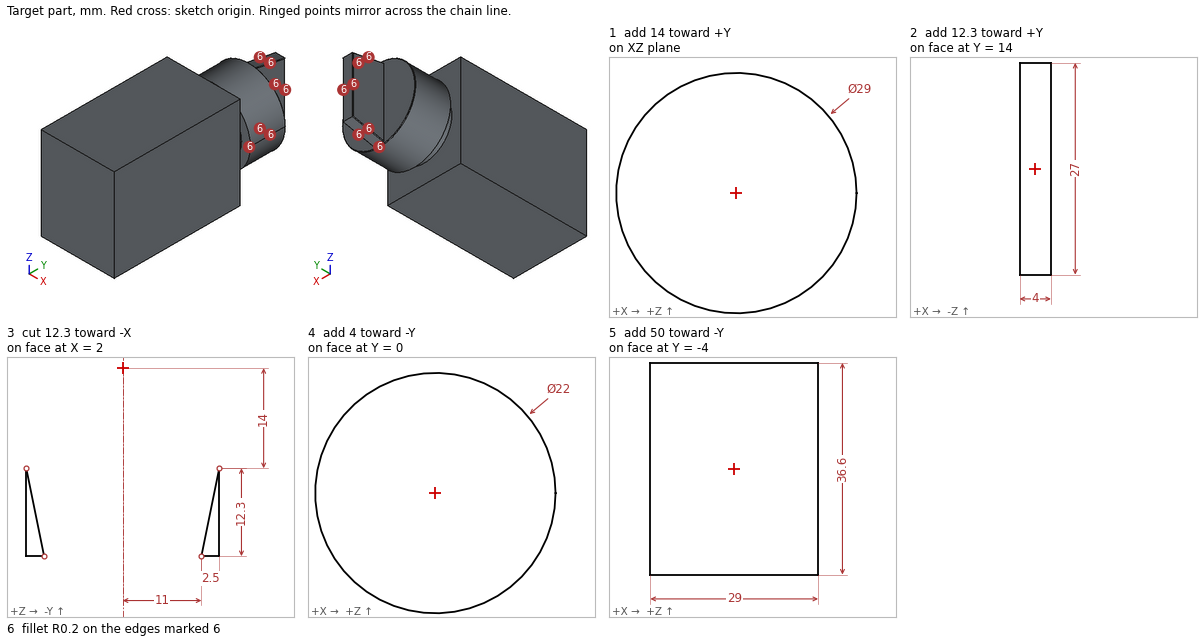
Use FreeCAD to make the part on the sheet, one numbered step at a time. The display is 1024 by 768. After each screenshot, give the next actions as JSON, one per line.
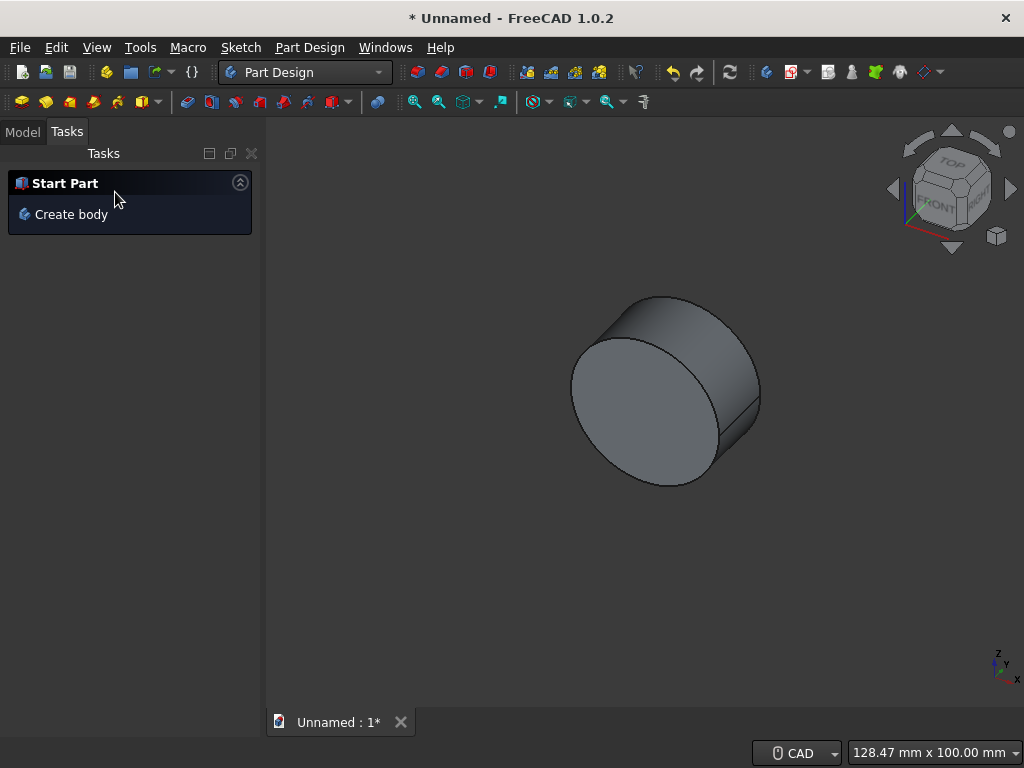
{"action": "left_click", "coordinate": [416, 102]}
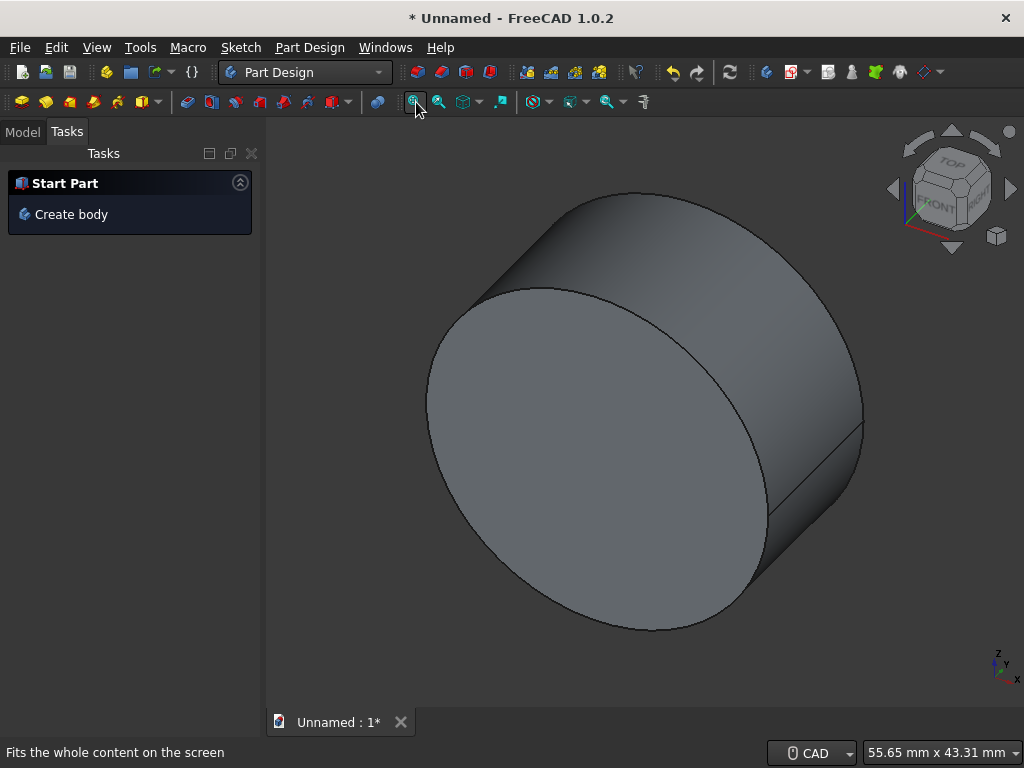
{"action": "key", "text": "4"}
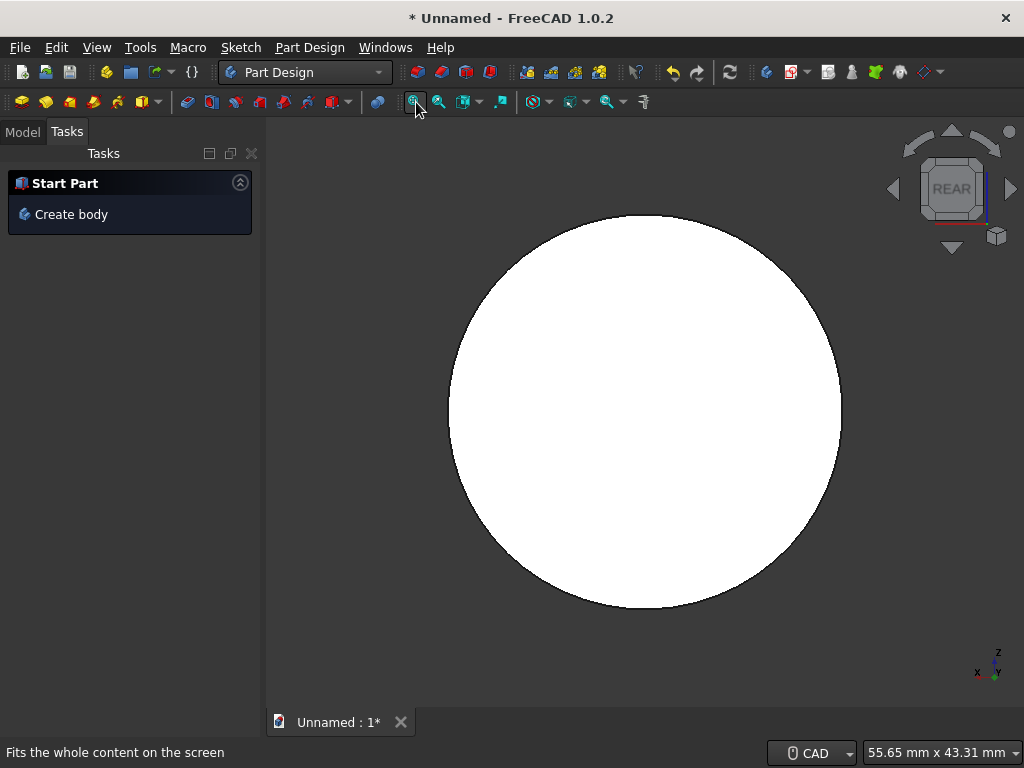
{"action": "left_click", "coordinate": [645, 411]}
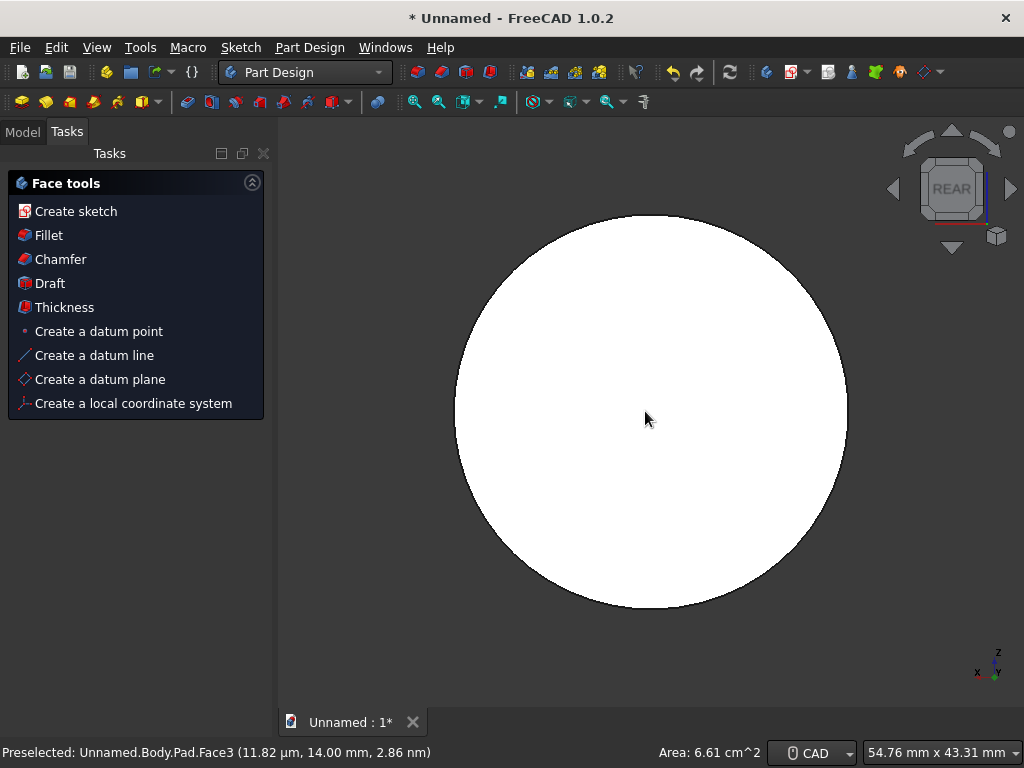
{"action": "left_click", "coordinate": [792, 72]}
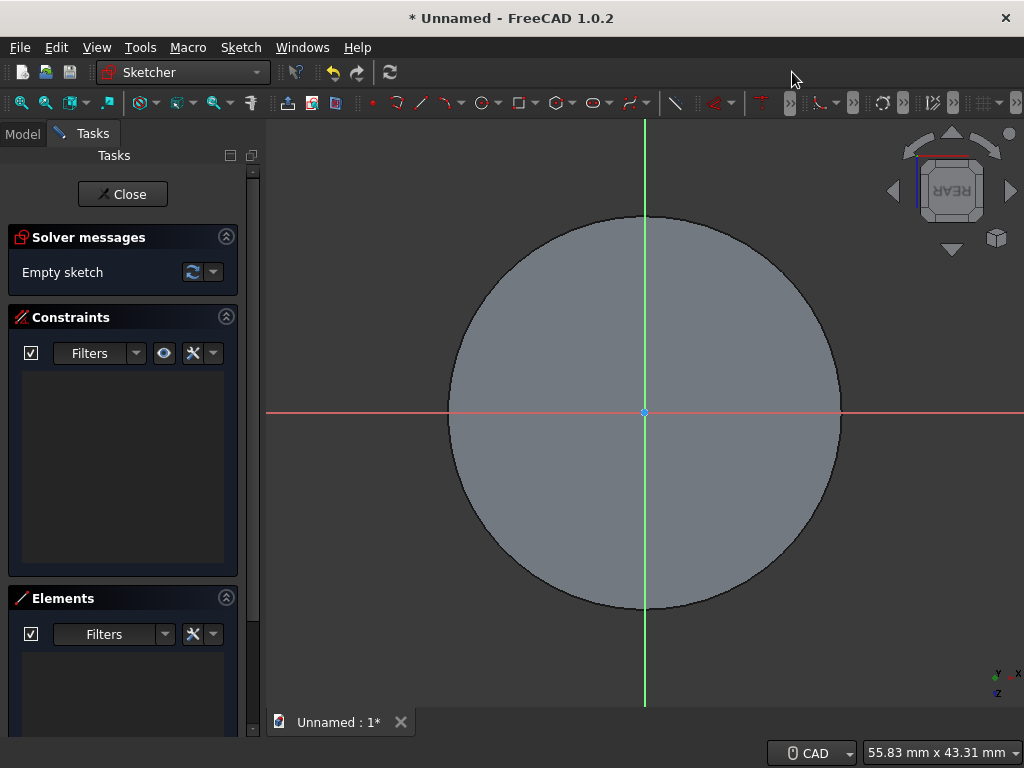
{"action": "left_click", "coordinate": [538, 104]}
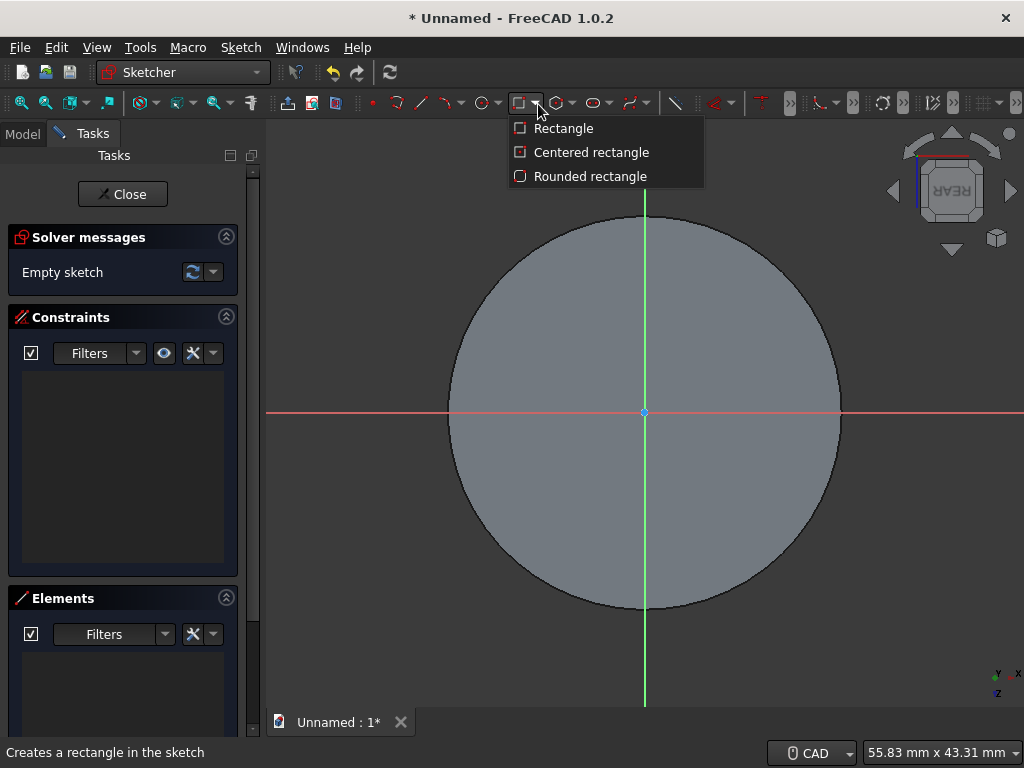
{"action": "left_click", "coordinate": [606, 152]}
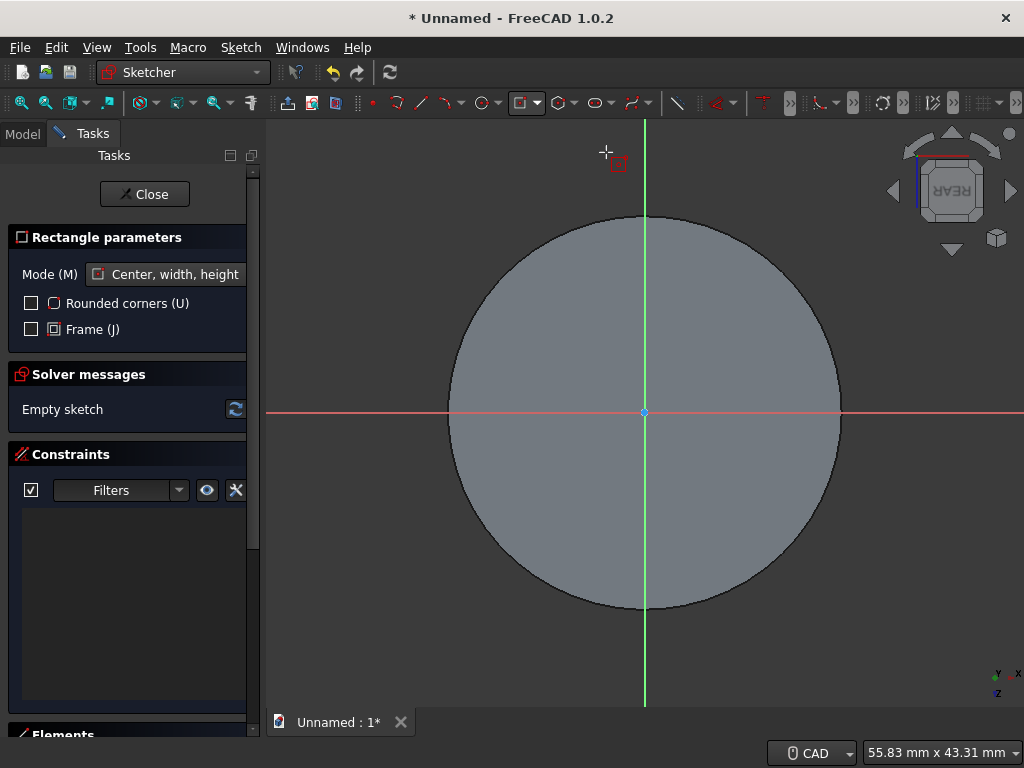
{"action": "left_click", "coordinate": [645, 413]}
{"action": "mouse_move", "coordinate": [672, 230]}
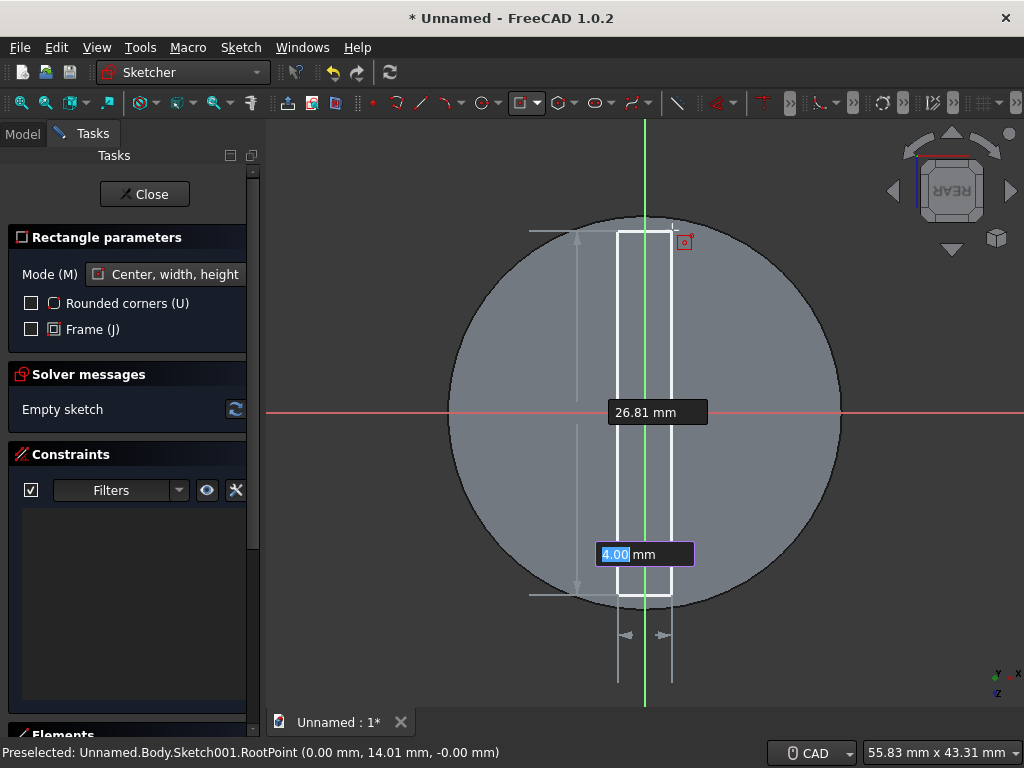
{"action": "type", "text": "4"}
{"action": "key", "text": "Tab"}
{"action": "type", "text": "27"}
{"action": "key", "text": "Return"}
{"action": "key", "text": "Escape"}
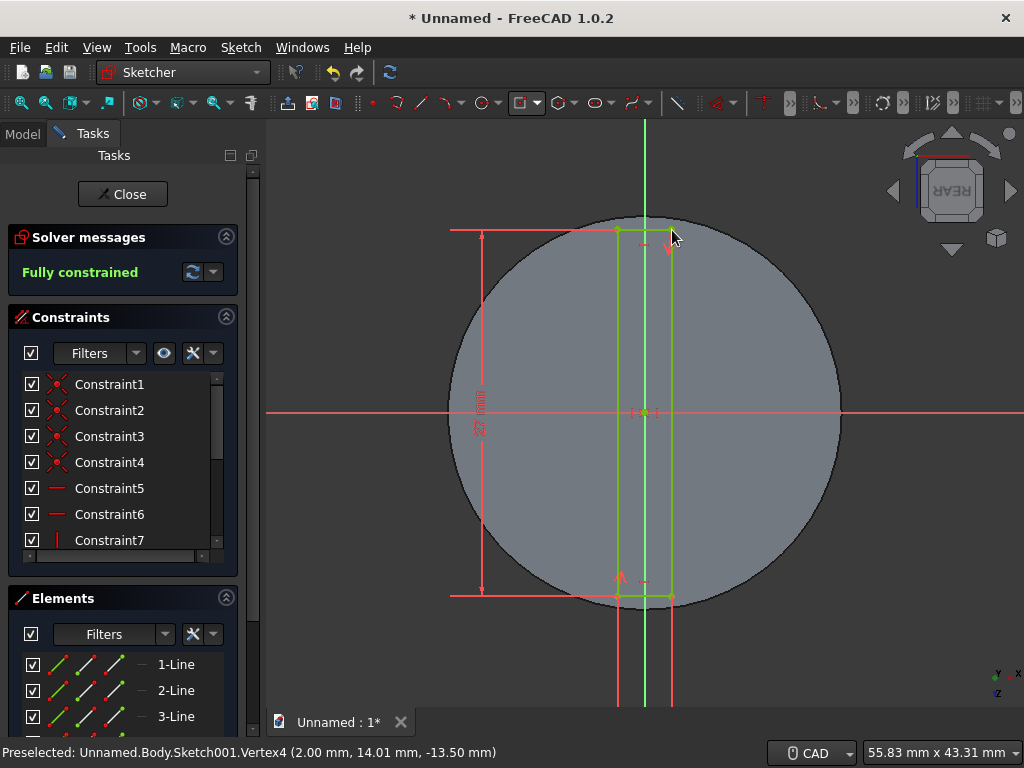
{"action": "left_click", "coordinate": [123, 194]}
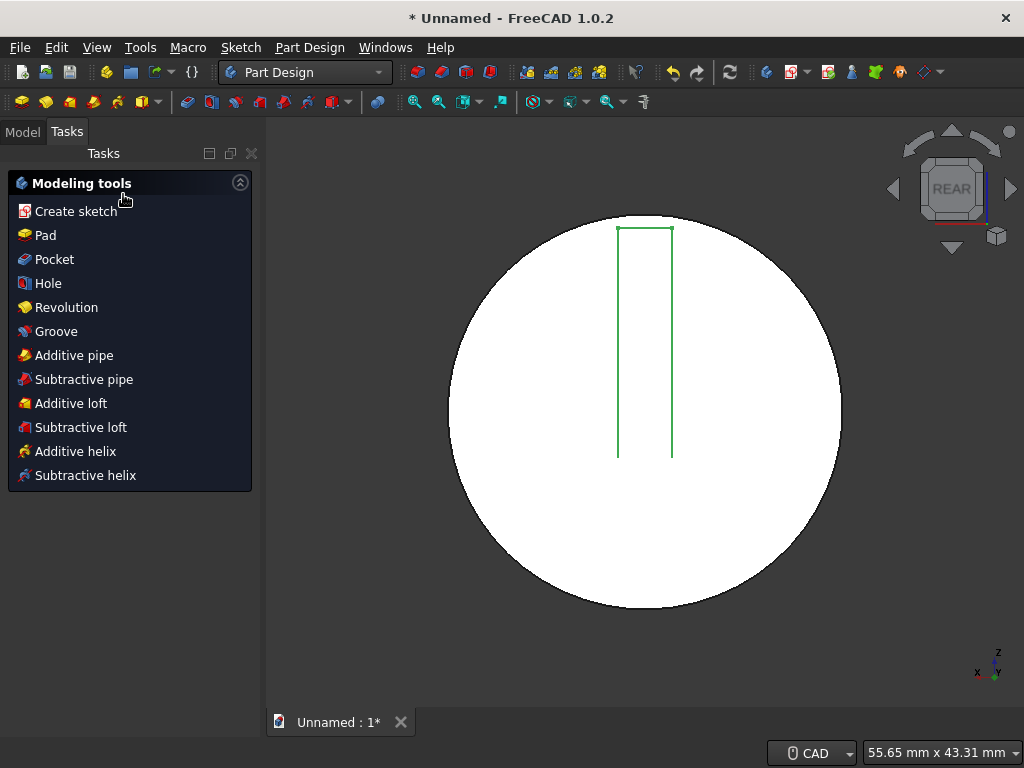
{"action": "left_click", "coordinate": [22, 102]}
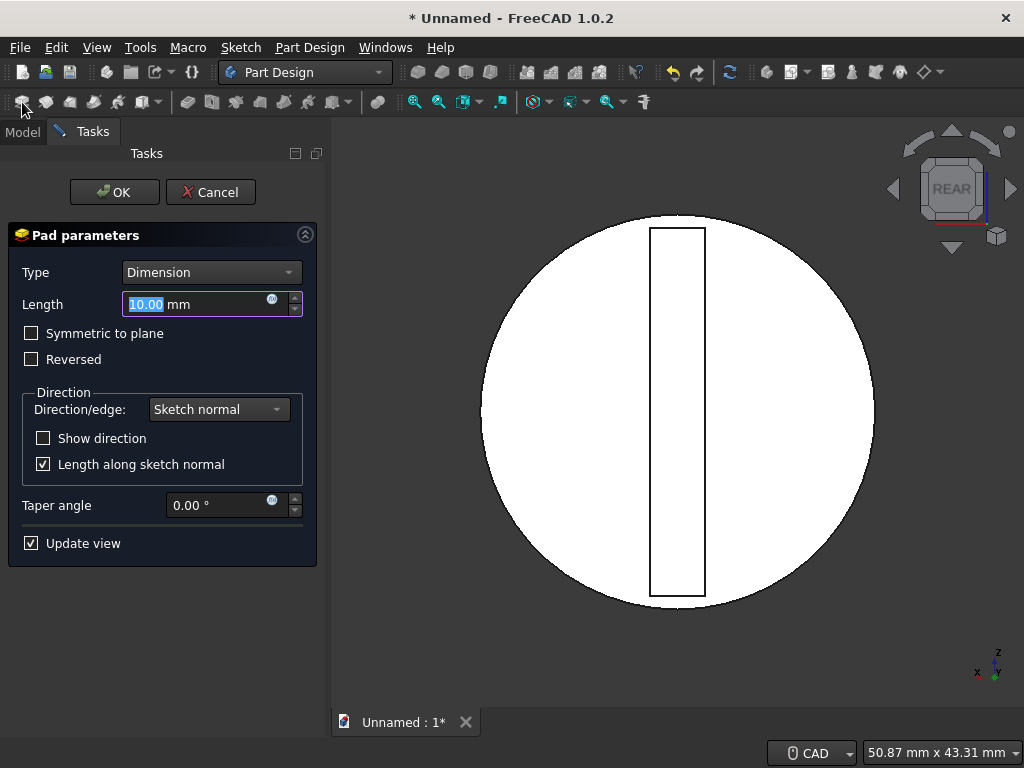
{"action": "type", "text": "12.3"}
{"action": "key", "text": "Tab"}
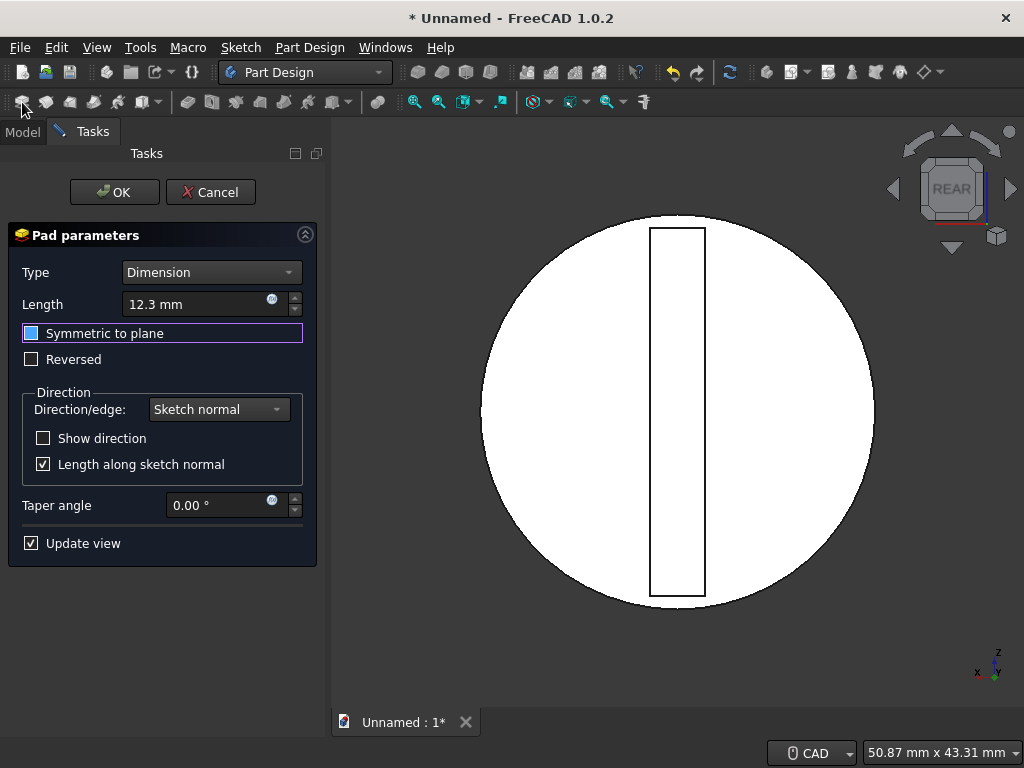
{"action": "left_click", "coordinate": [115, 192]}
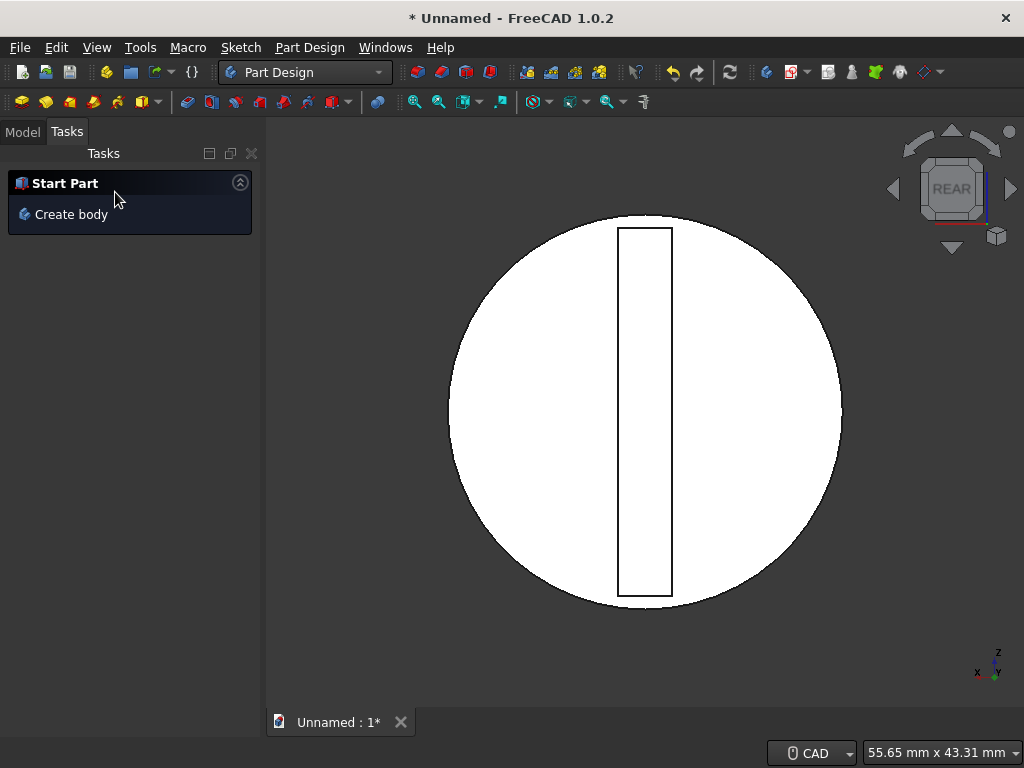
{"action": "key", "text": "0"}